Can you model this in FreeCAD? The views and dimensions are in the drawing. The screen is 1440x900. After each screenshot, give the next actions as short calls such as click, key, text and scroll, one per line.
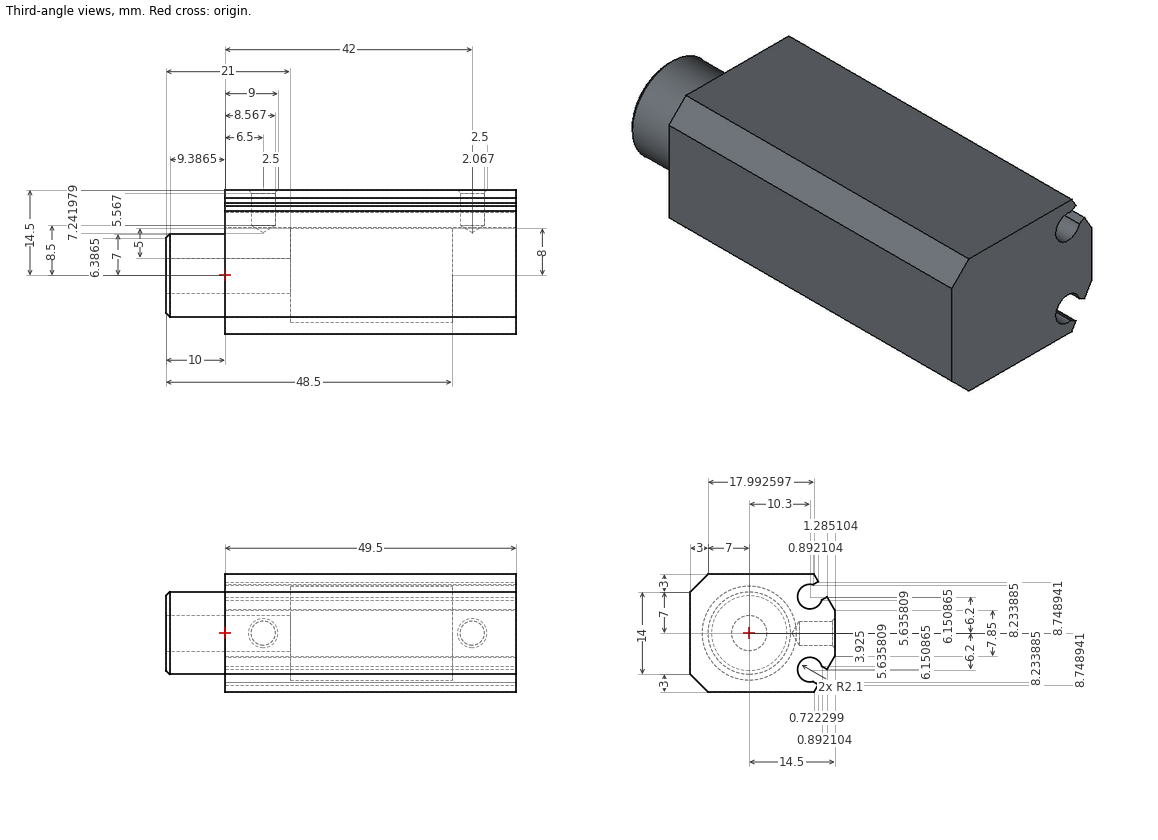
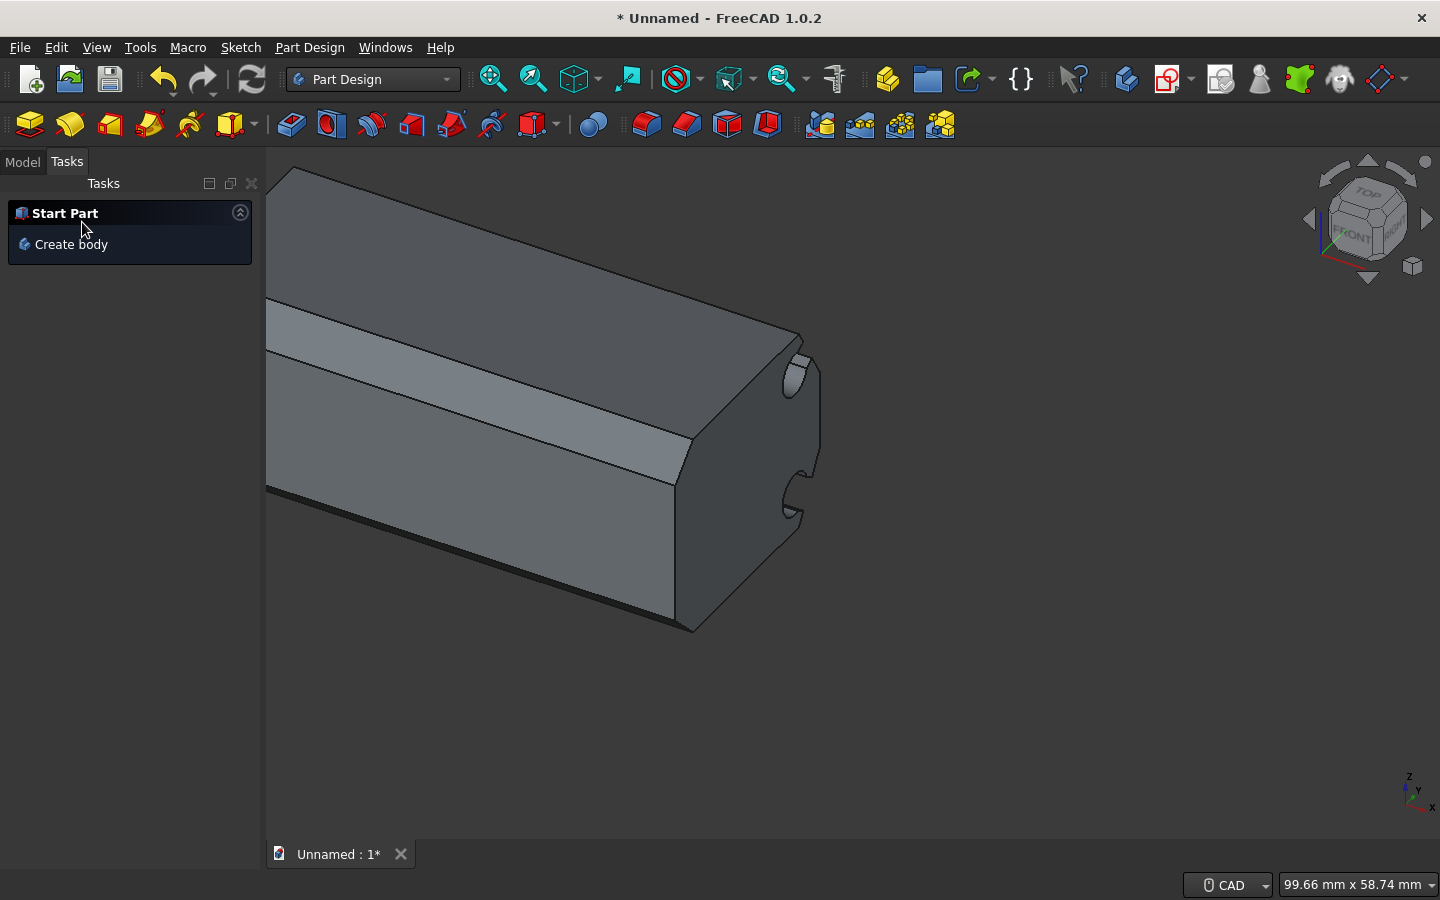
click(494, 80)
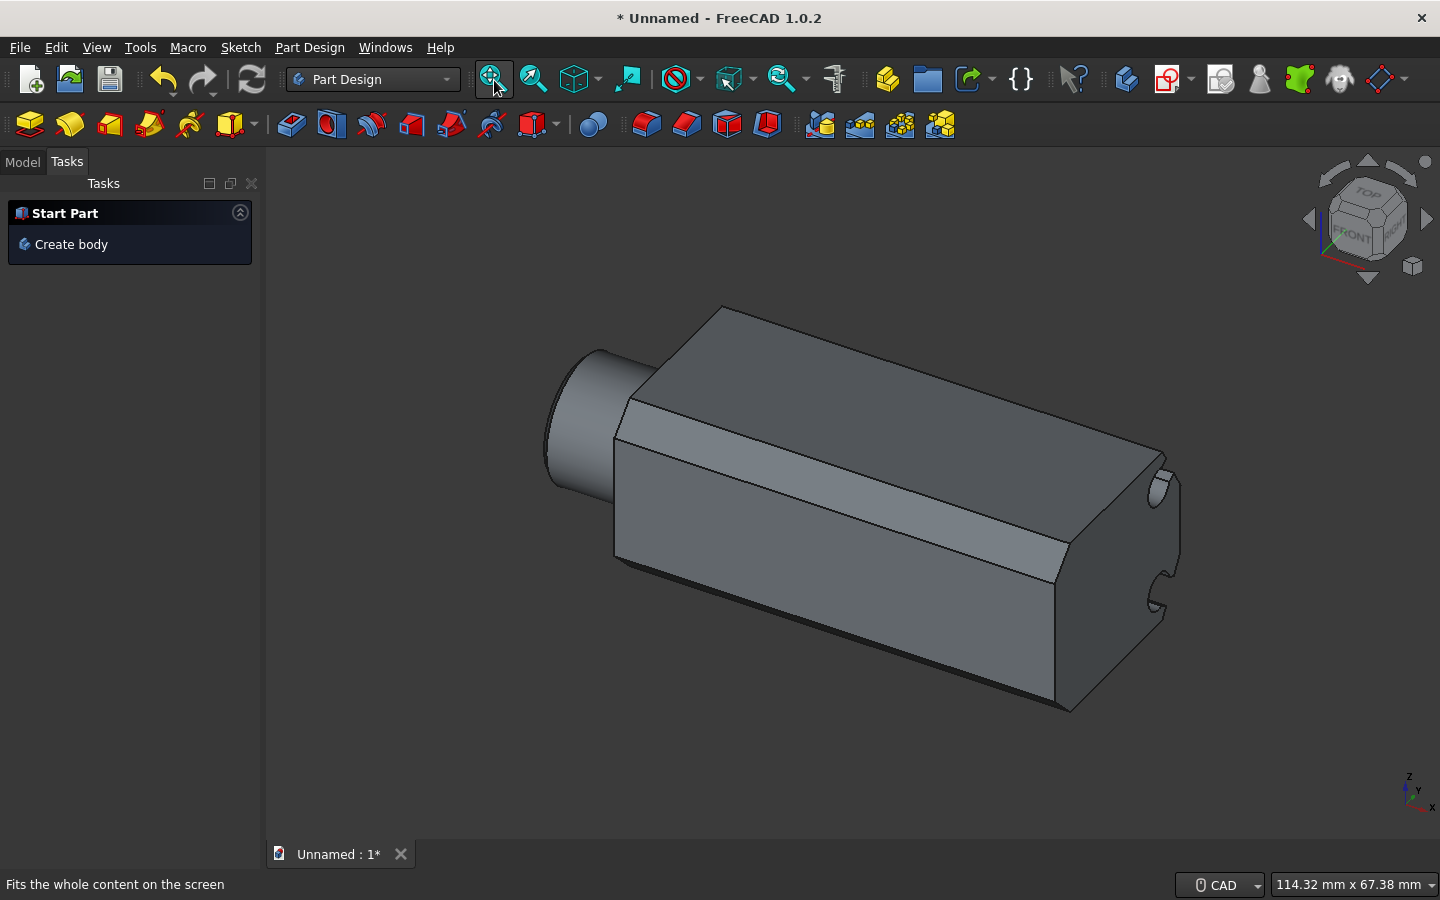
click(1168, 80)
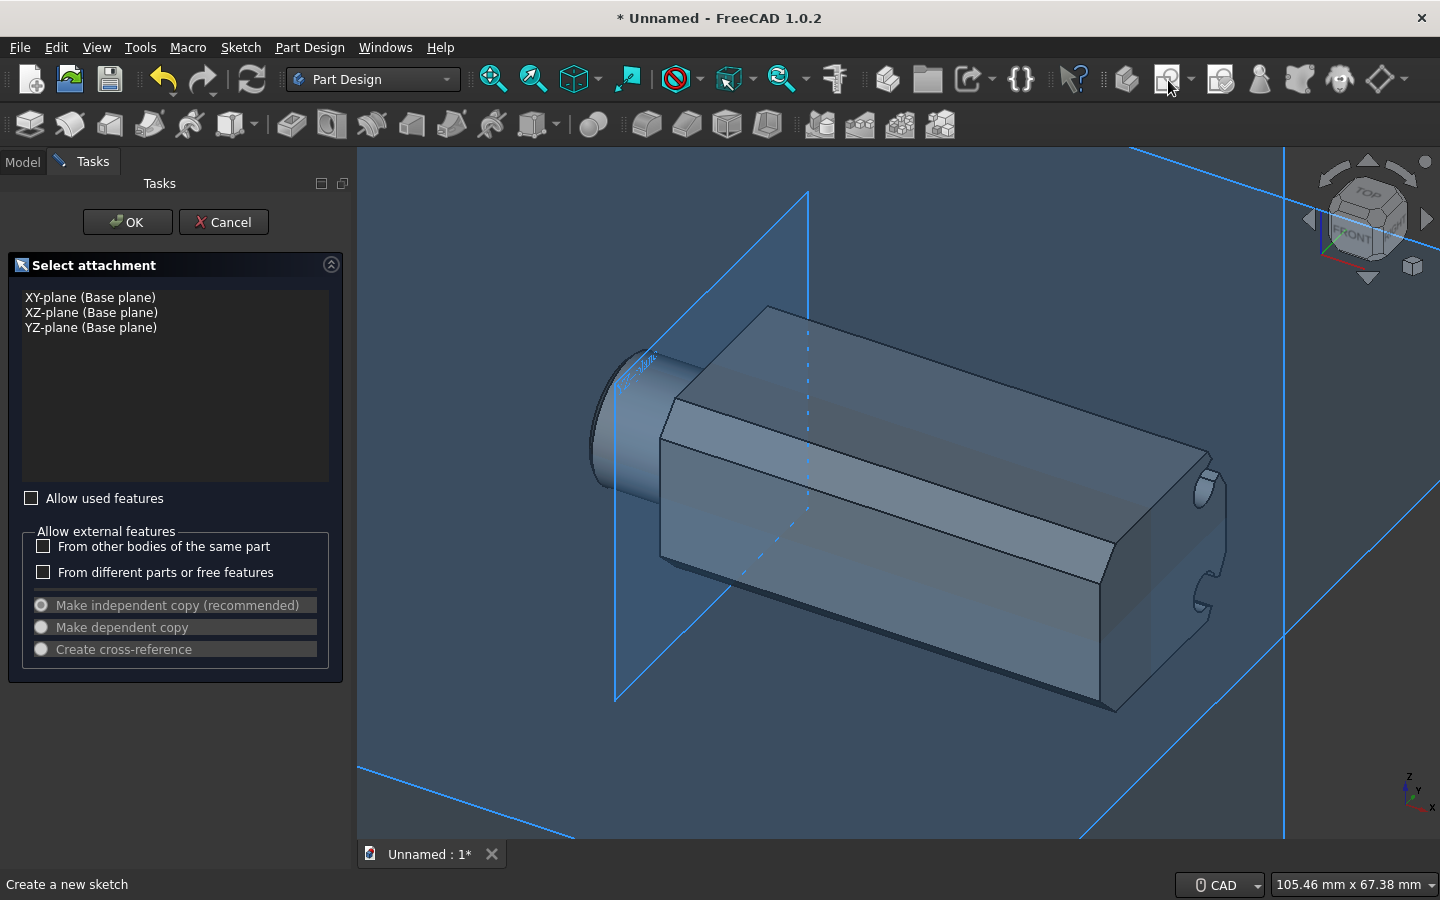
click(82, 298)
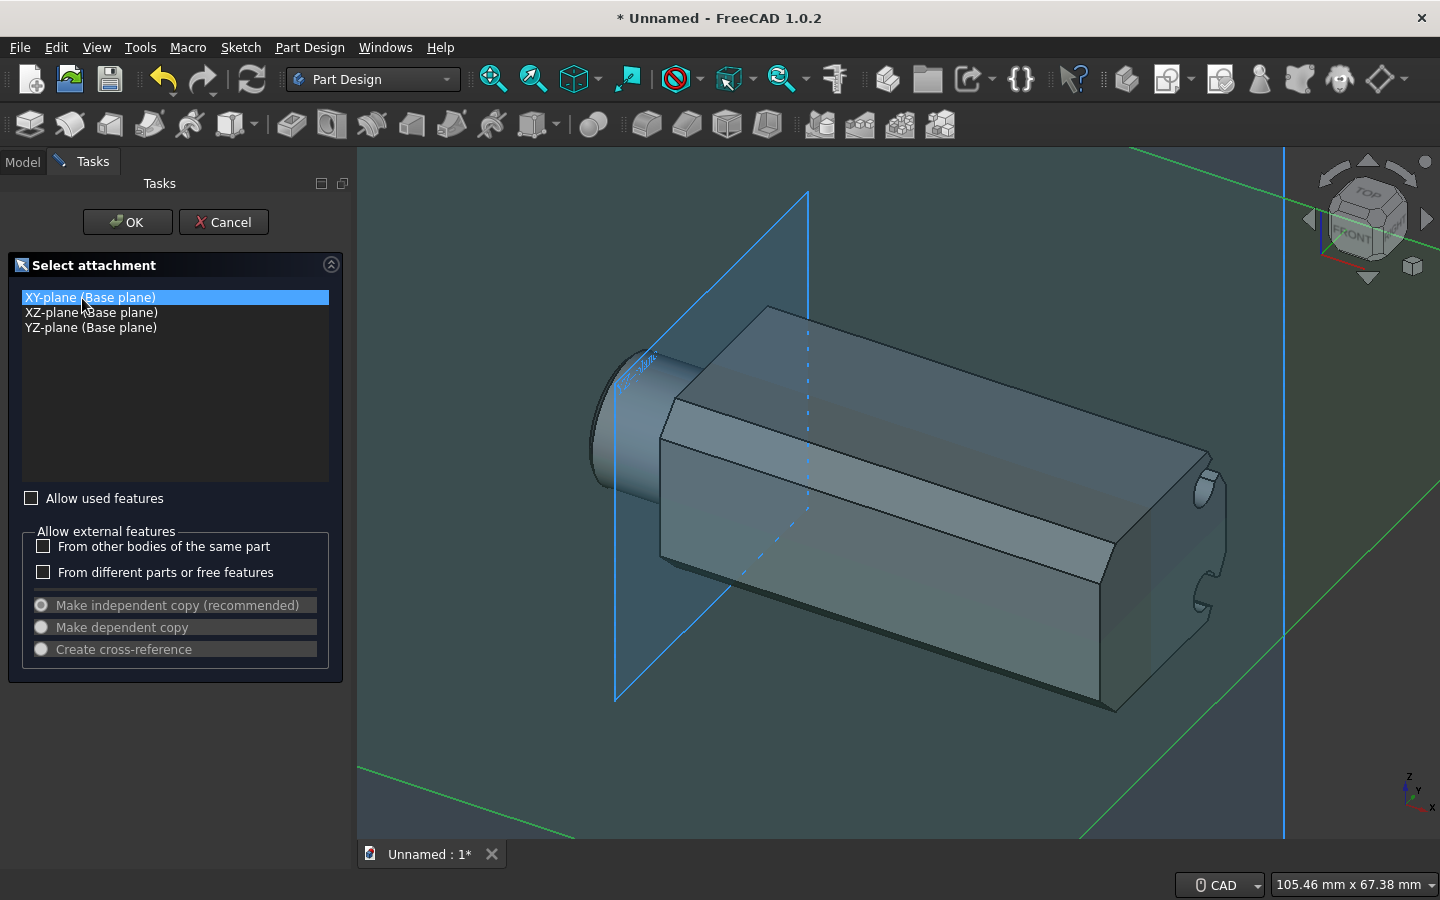
click(128, 222)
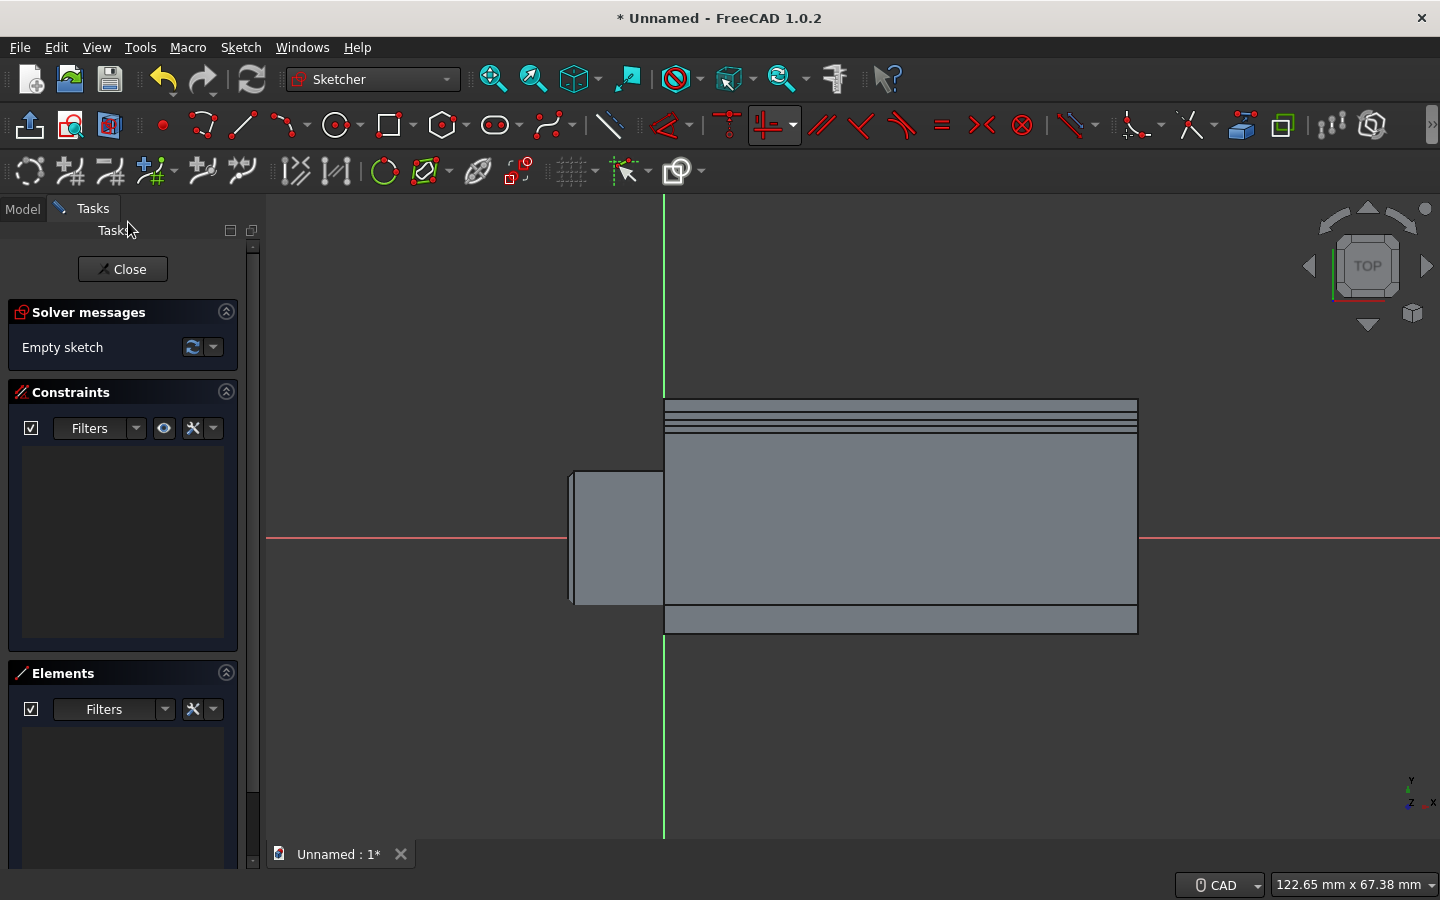
click(110, 126)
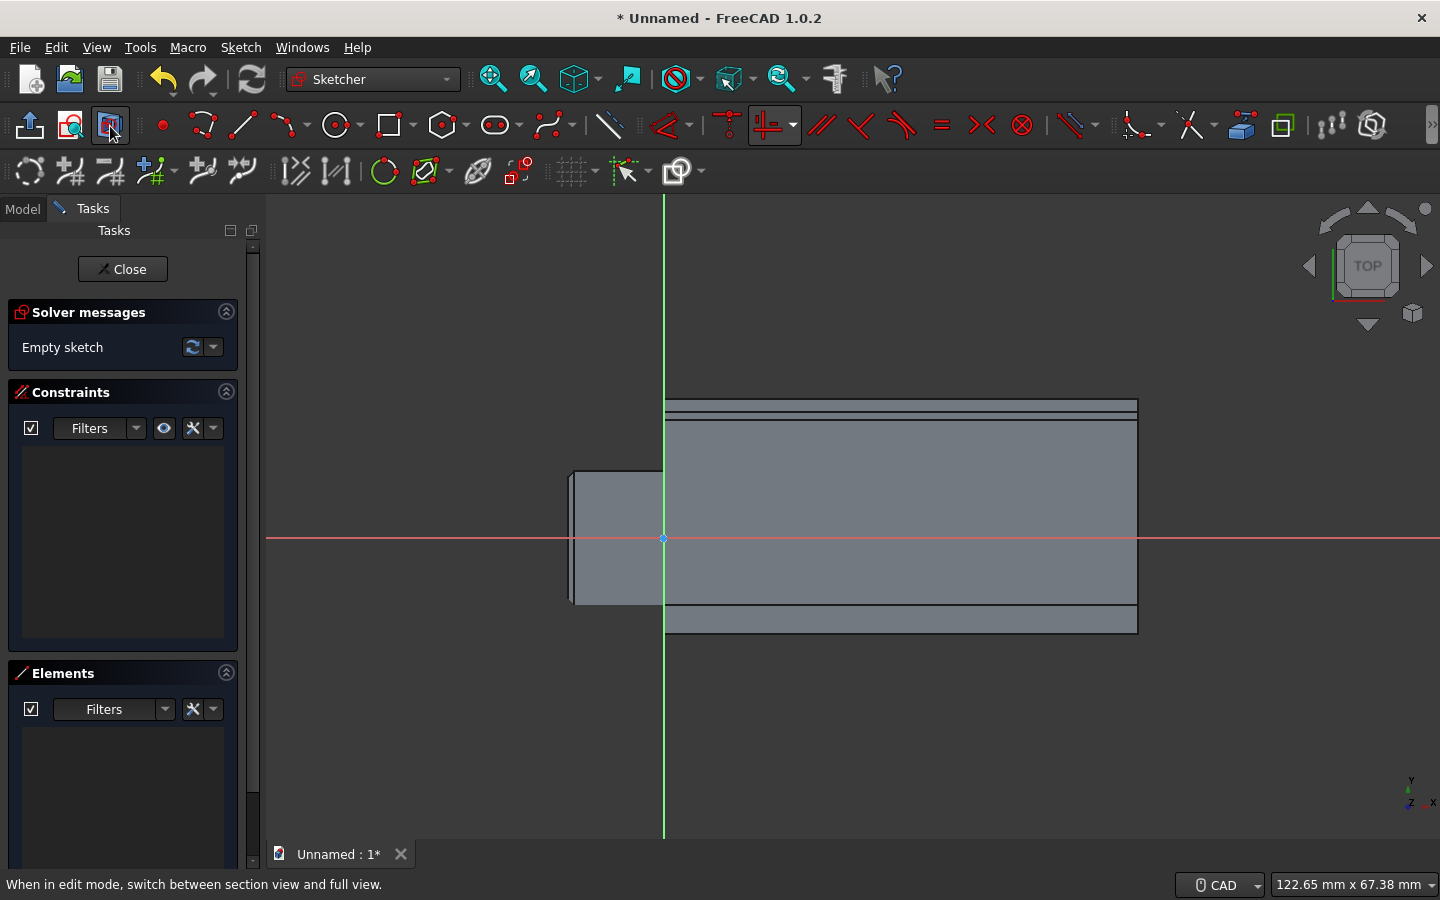
scroll(833, 466, up, 2)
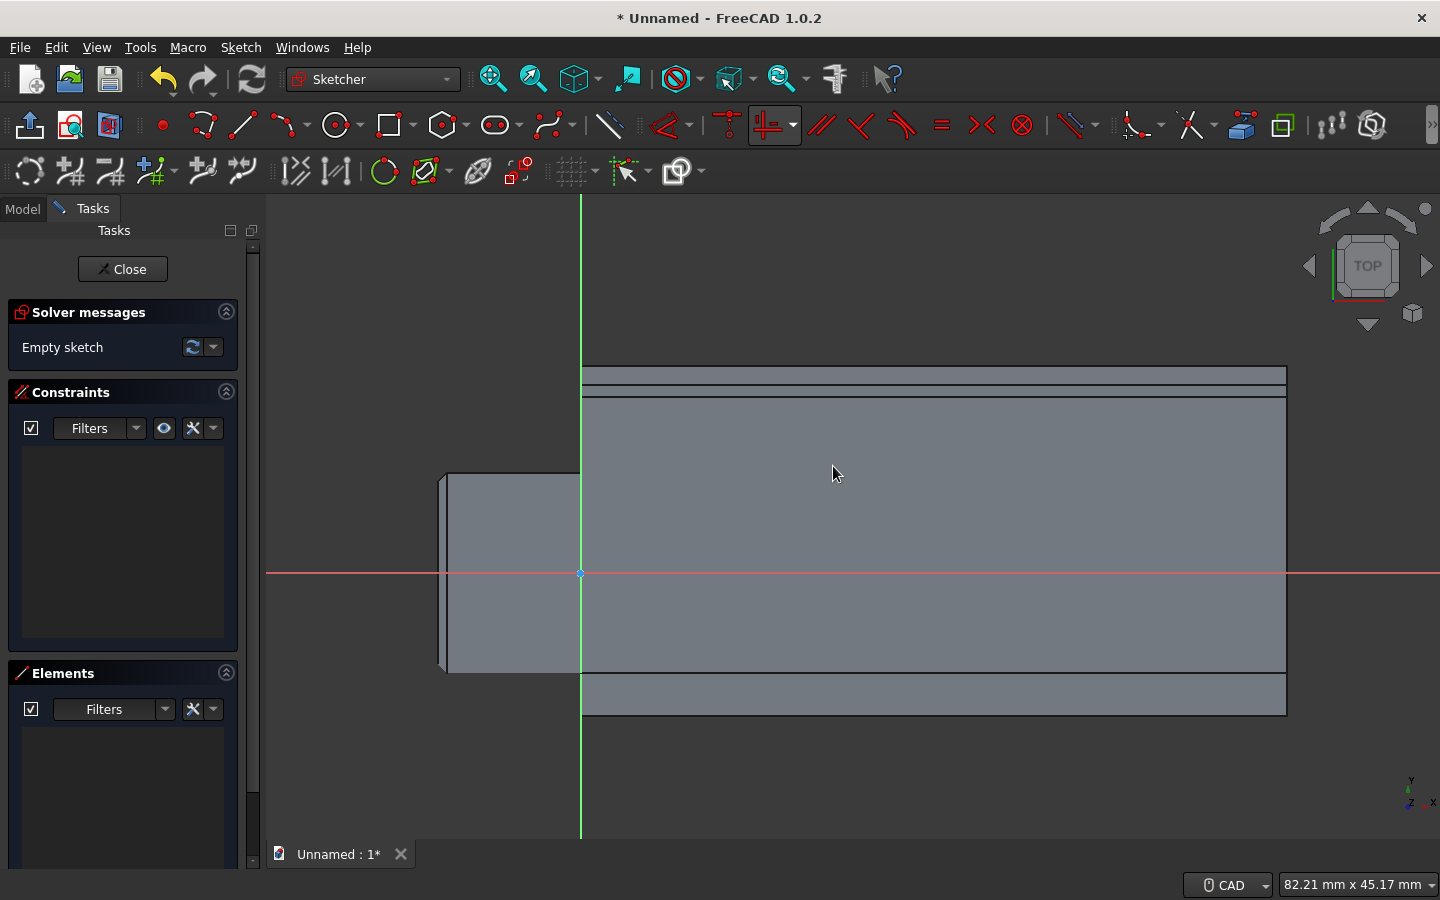
click(204, 126)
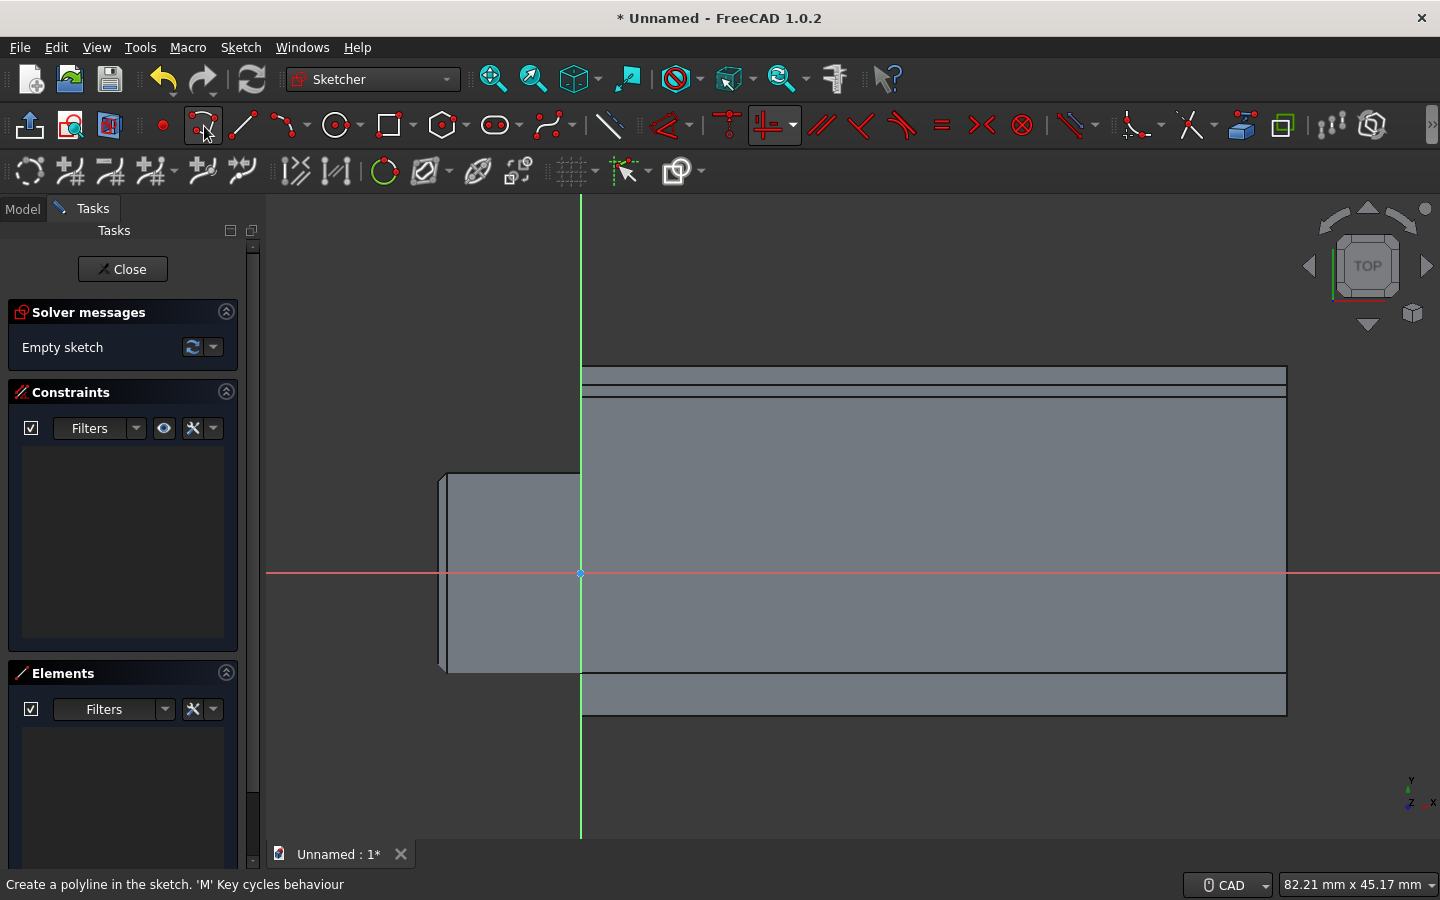
click(438, 573)
click(1130, 564)
click(1130, 459)
click(738, 459)
click(738, 530)
click(438, 530)
click(438, 573)
key(Escape)
key(Escape)